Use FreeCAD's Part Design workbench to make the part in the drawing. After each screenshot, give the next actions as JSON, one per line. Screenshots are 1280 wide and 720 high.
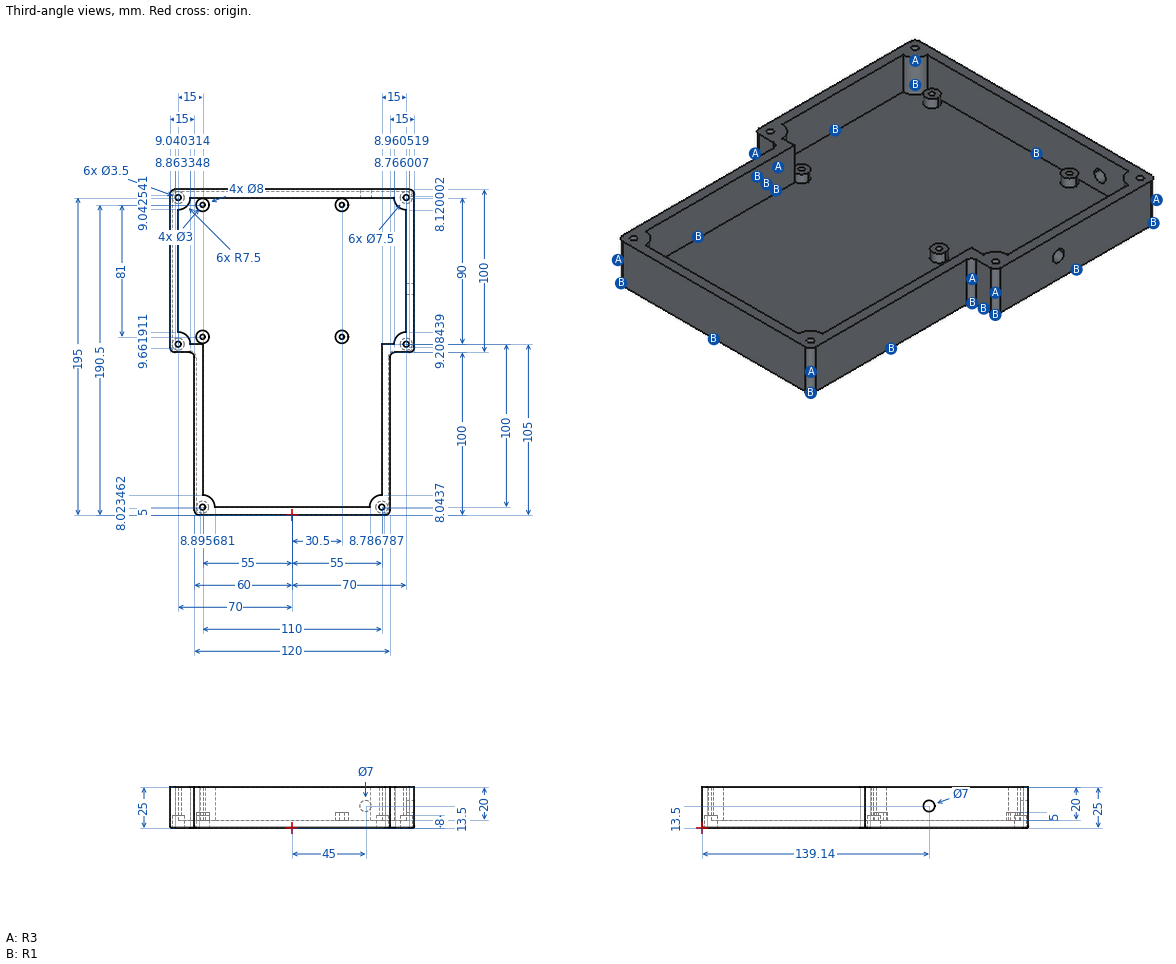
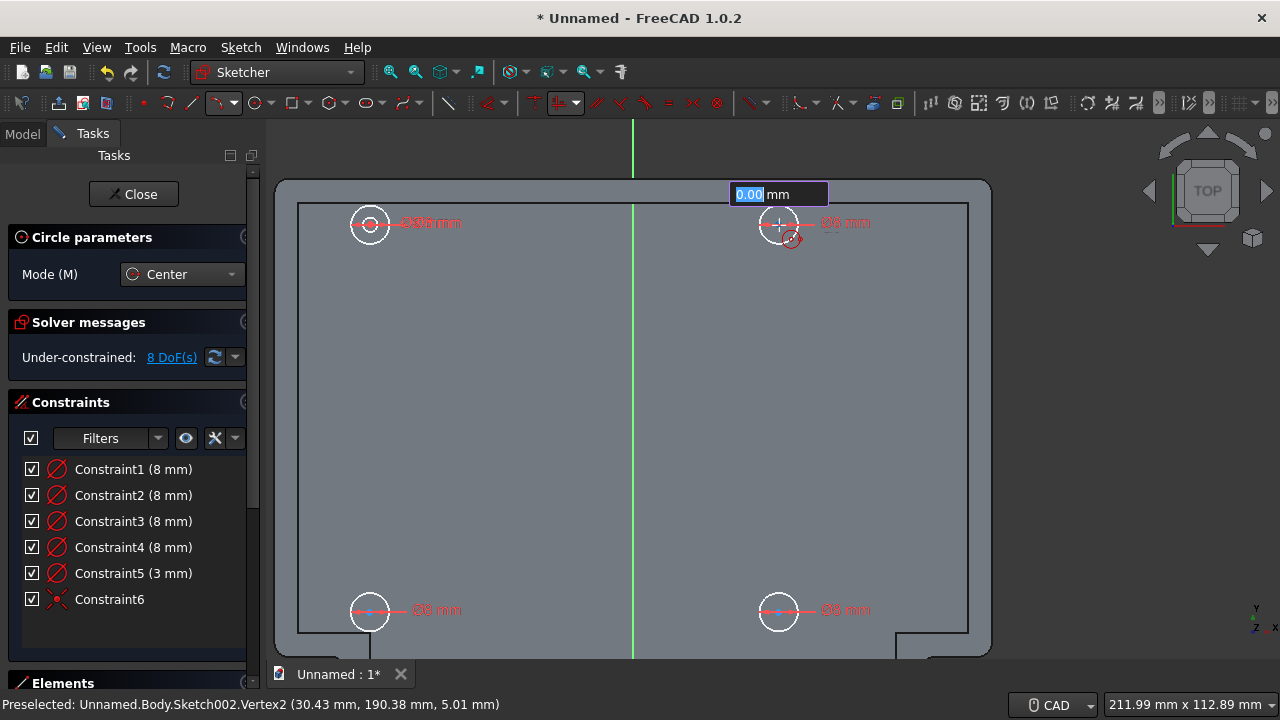
{"action": "scroll", "coordinate": [781, 217], "scroll_direction": "up", "scroll_amount": 4}
{"action": "mouse_move", "coordinate": [781, 217]}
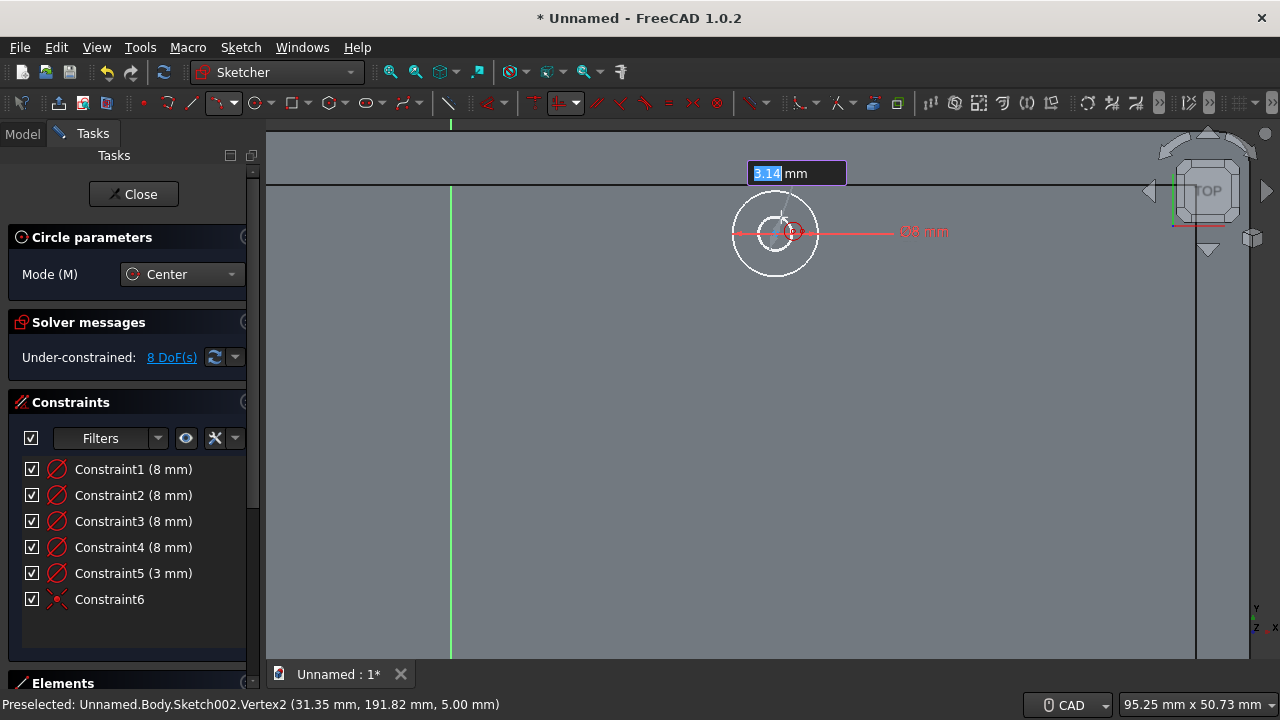
{"action": "type", "text": "3"}
{"action": "key", "text": "Return"}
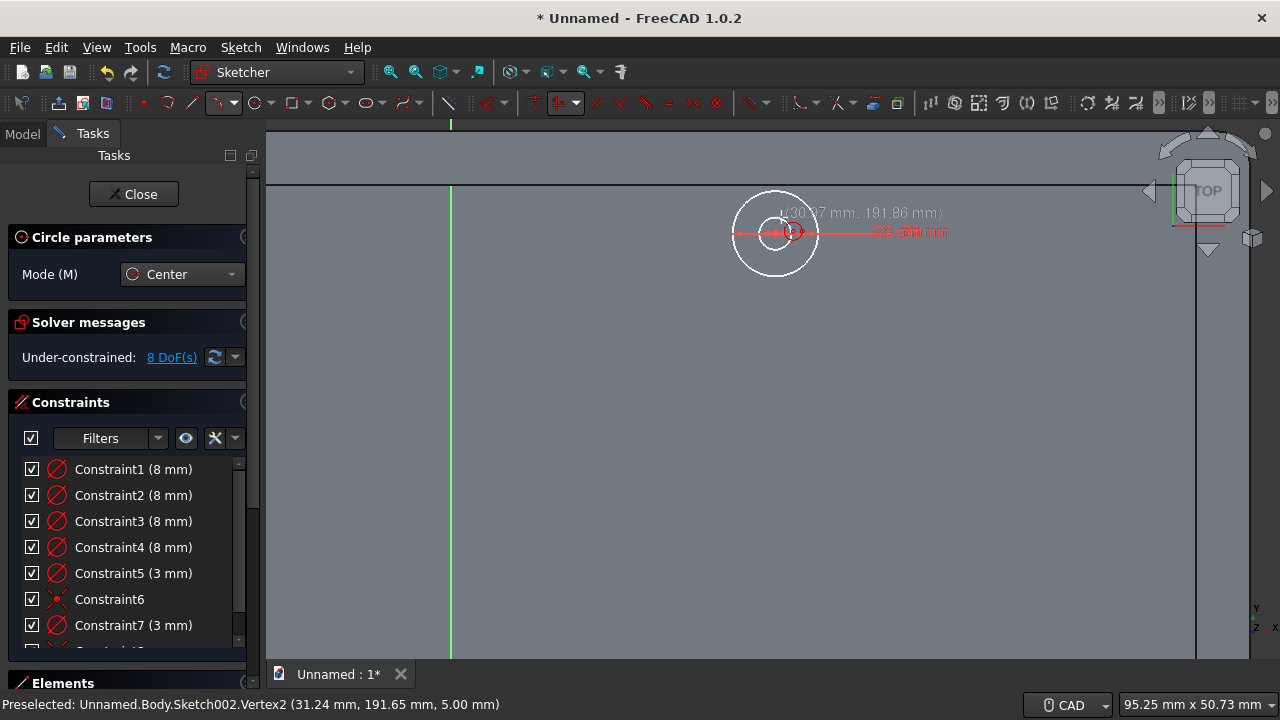
{"action": "scroll", "coordinate": [780, 223], "scroll_direction": "down", "scroll_amount": 9}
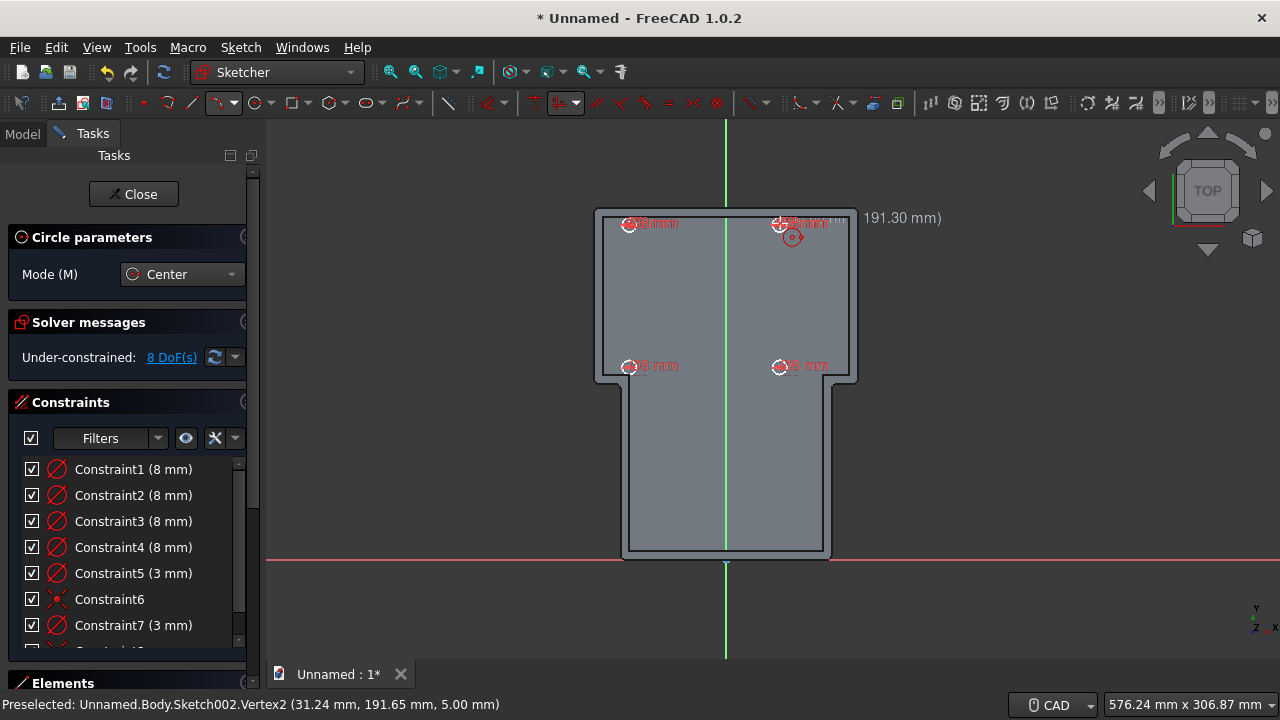
{"action": "scroll", "coordinate": [629, 367], "scroll_direction": "up", "scroll_amount": 11}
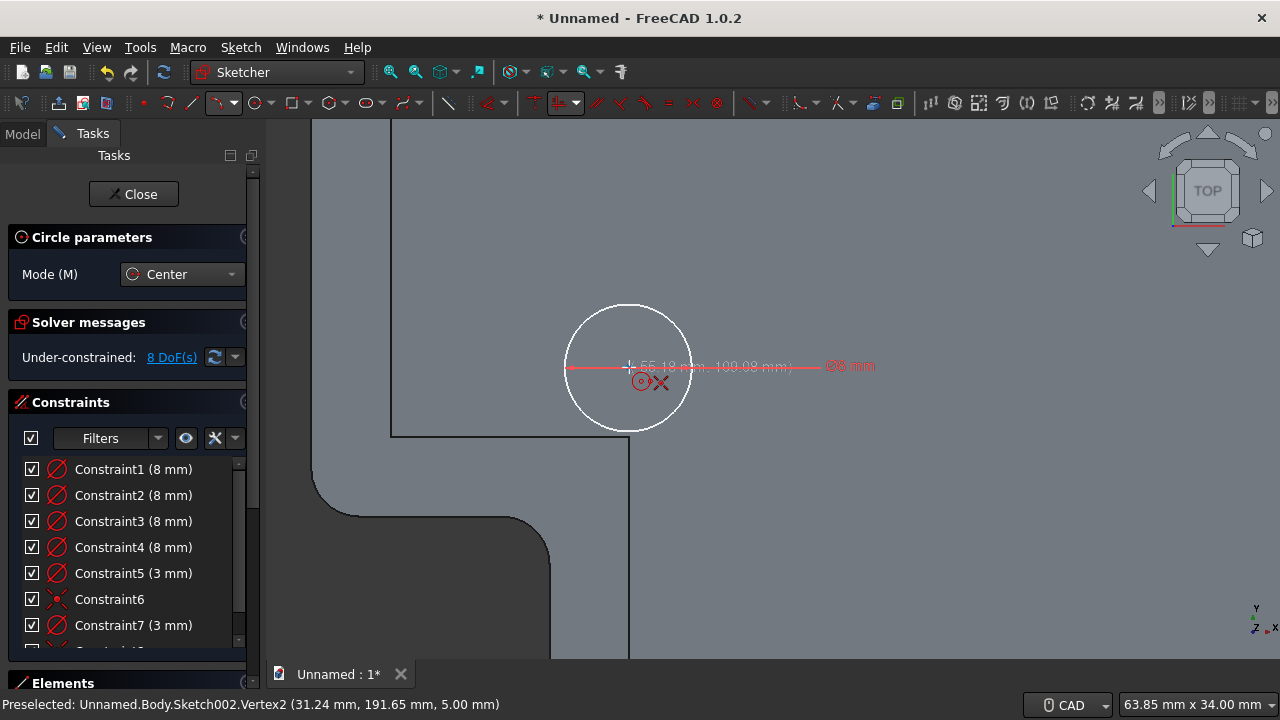
{"action": "scroll", "coordinate": [629, 368], "scroll_direction": "down", "scroll_amount": 11}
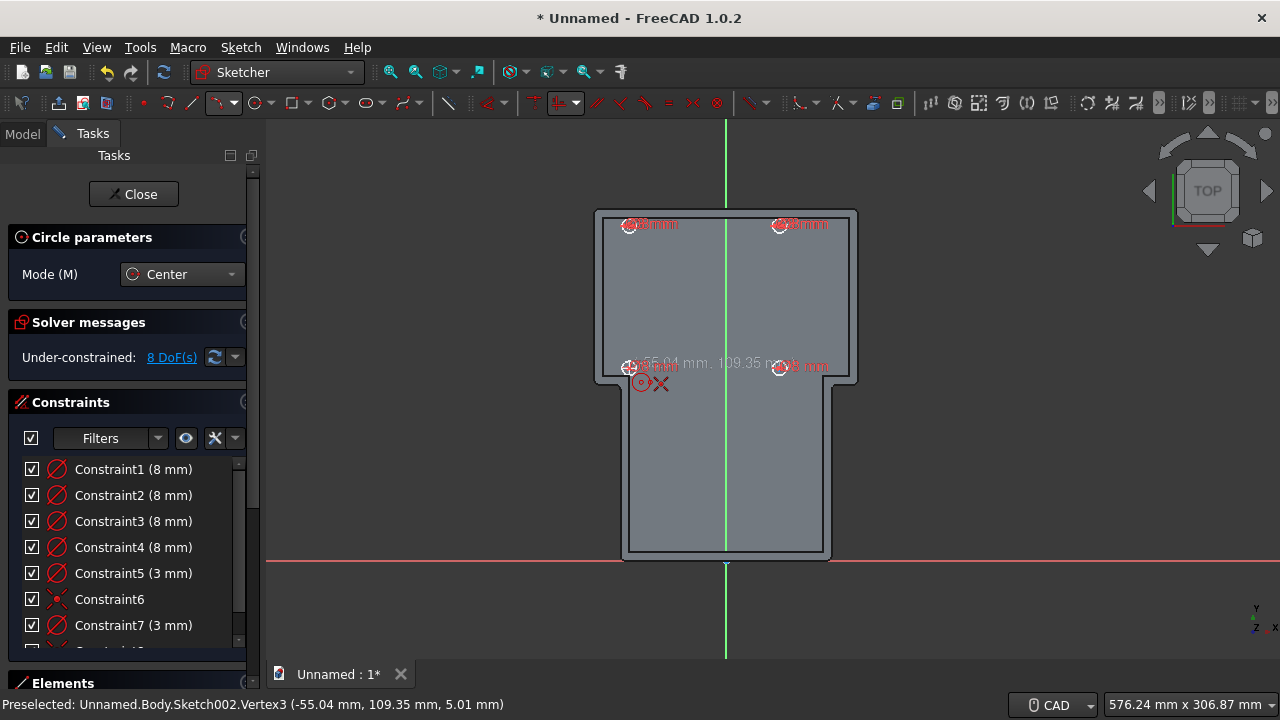
{"action": "scroll", "coordinate": [629, 368], "scroll_direction": "up", "scroll_amount": 5}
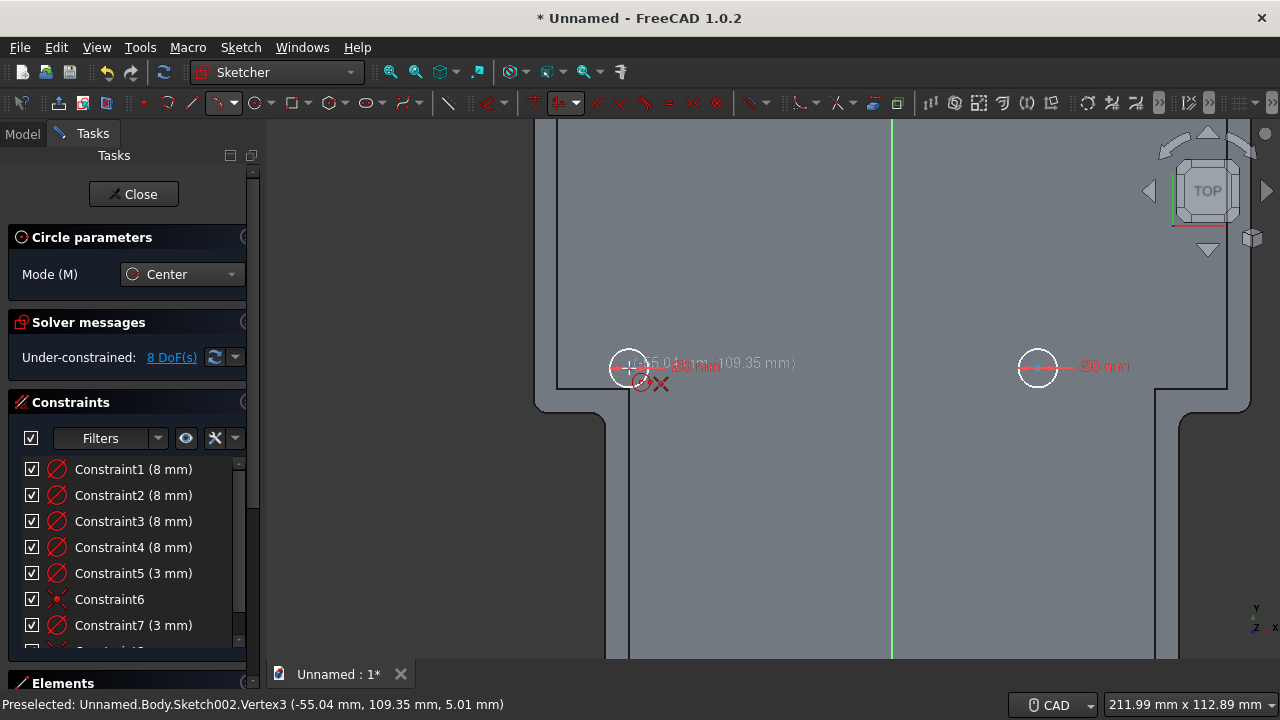
{"action": "left_click", "coordinate": [629, 368]}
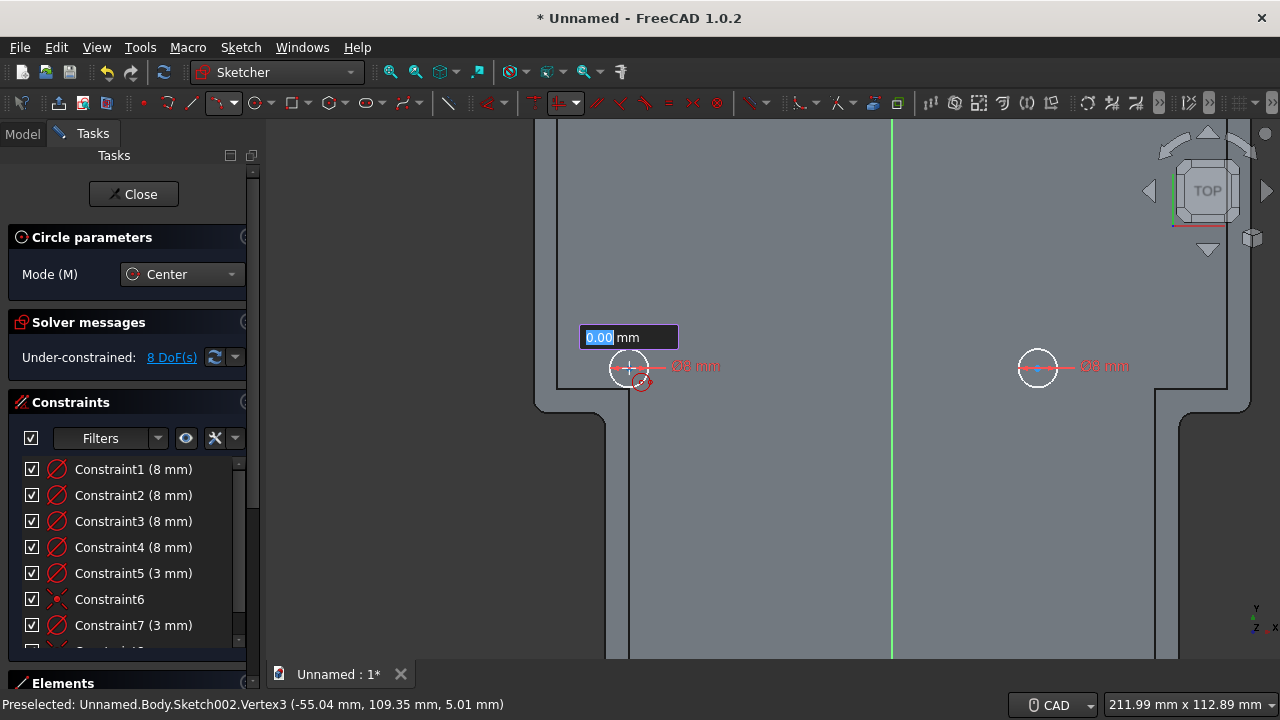
{"action": "scroll", "coordinate": [636, 365], "scroll_direction": "up", "scroll_amount": 4}
{"action": "mouse_move", "coordinate": [635, 365]}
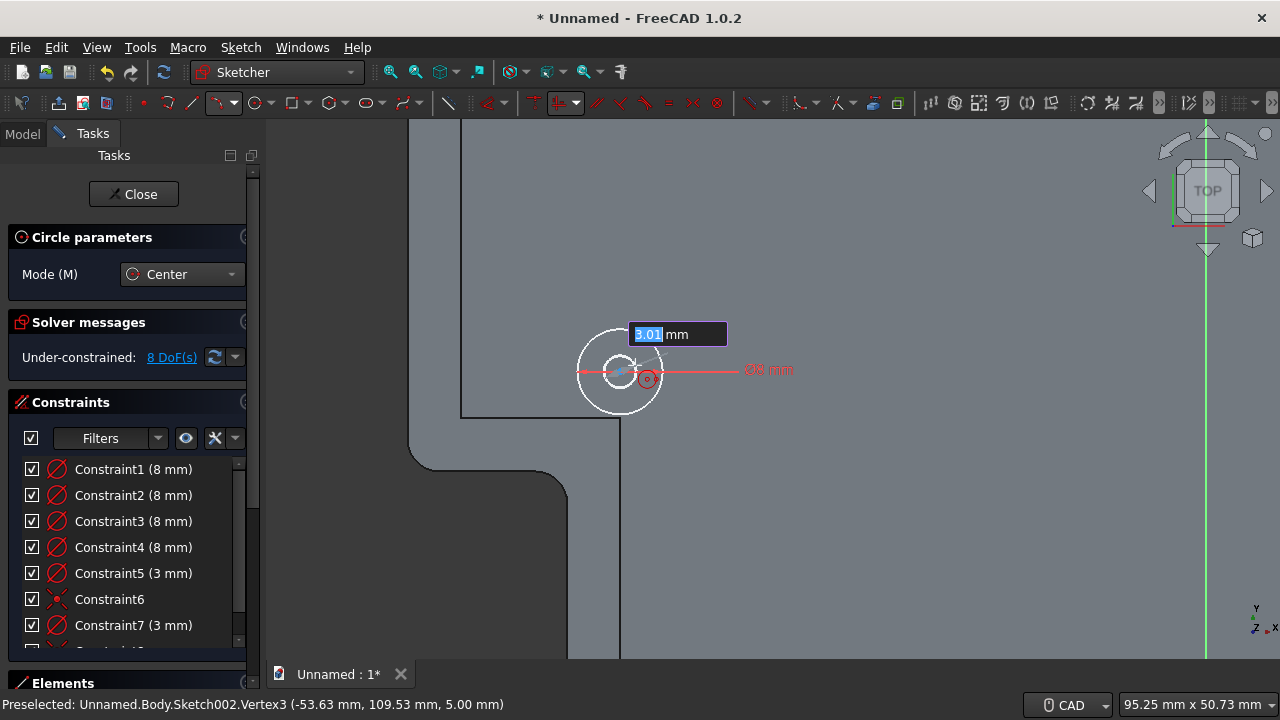
{"action": "type", "text": "3"}
{"action": "key", "text": "Return"}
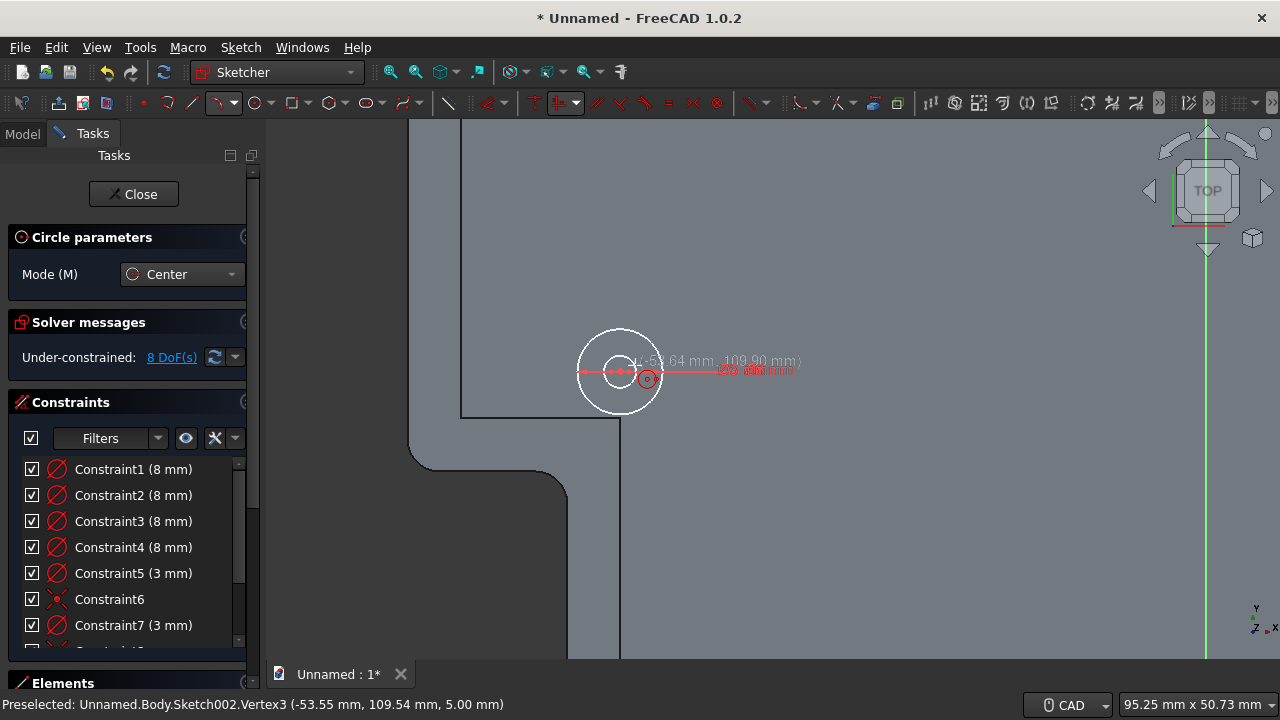
{"action": "scroll", "coordinate": [631, 367], "scroll_direction": "down", "scroll_amount": 9}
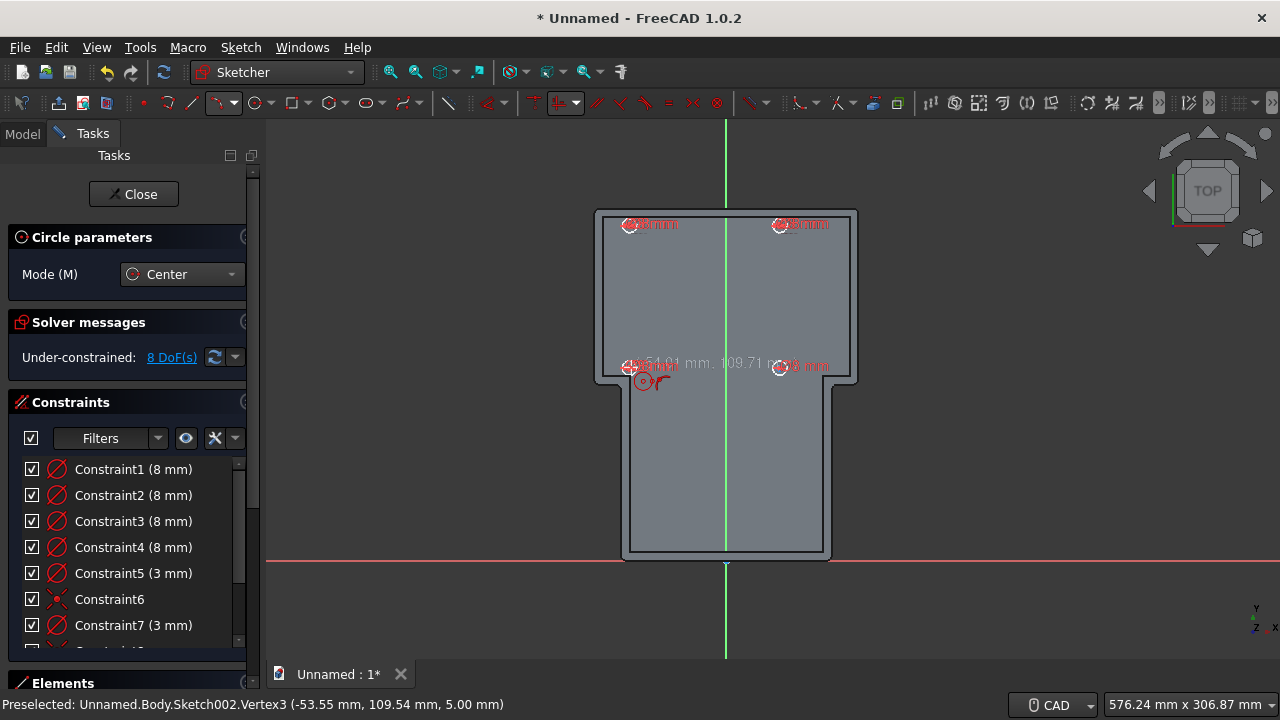
{"action": "scroll", "coordinate": [780, 368], "scroll_direction": "up", "scroll_amount": 11}